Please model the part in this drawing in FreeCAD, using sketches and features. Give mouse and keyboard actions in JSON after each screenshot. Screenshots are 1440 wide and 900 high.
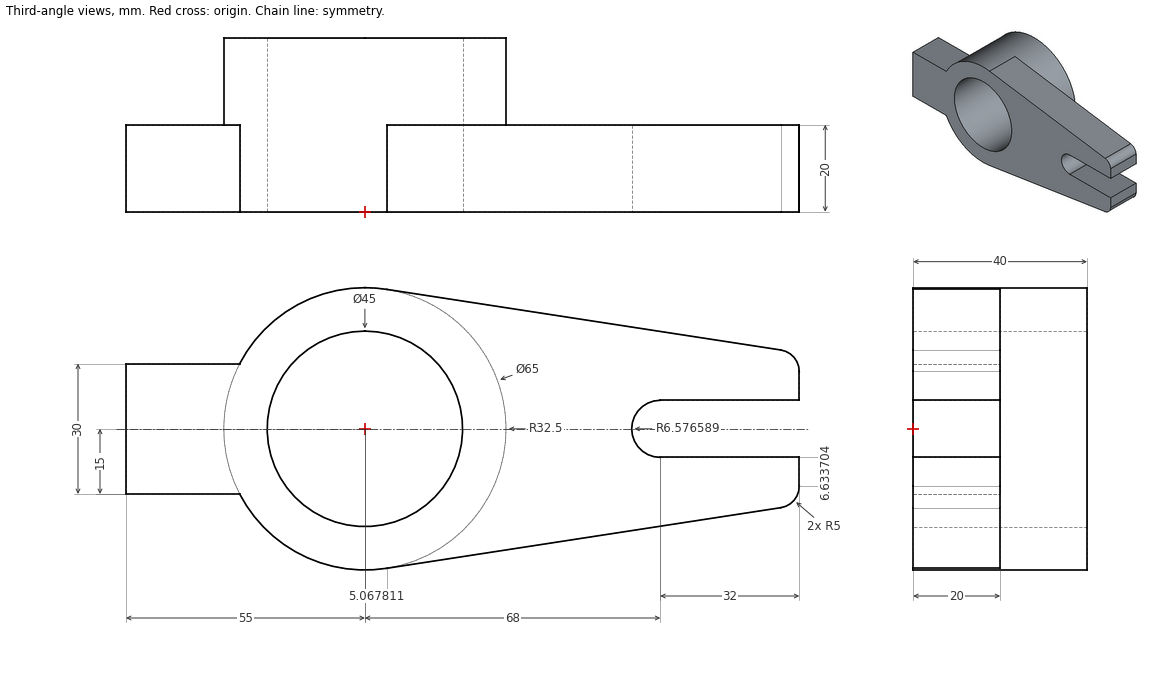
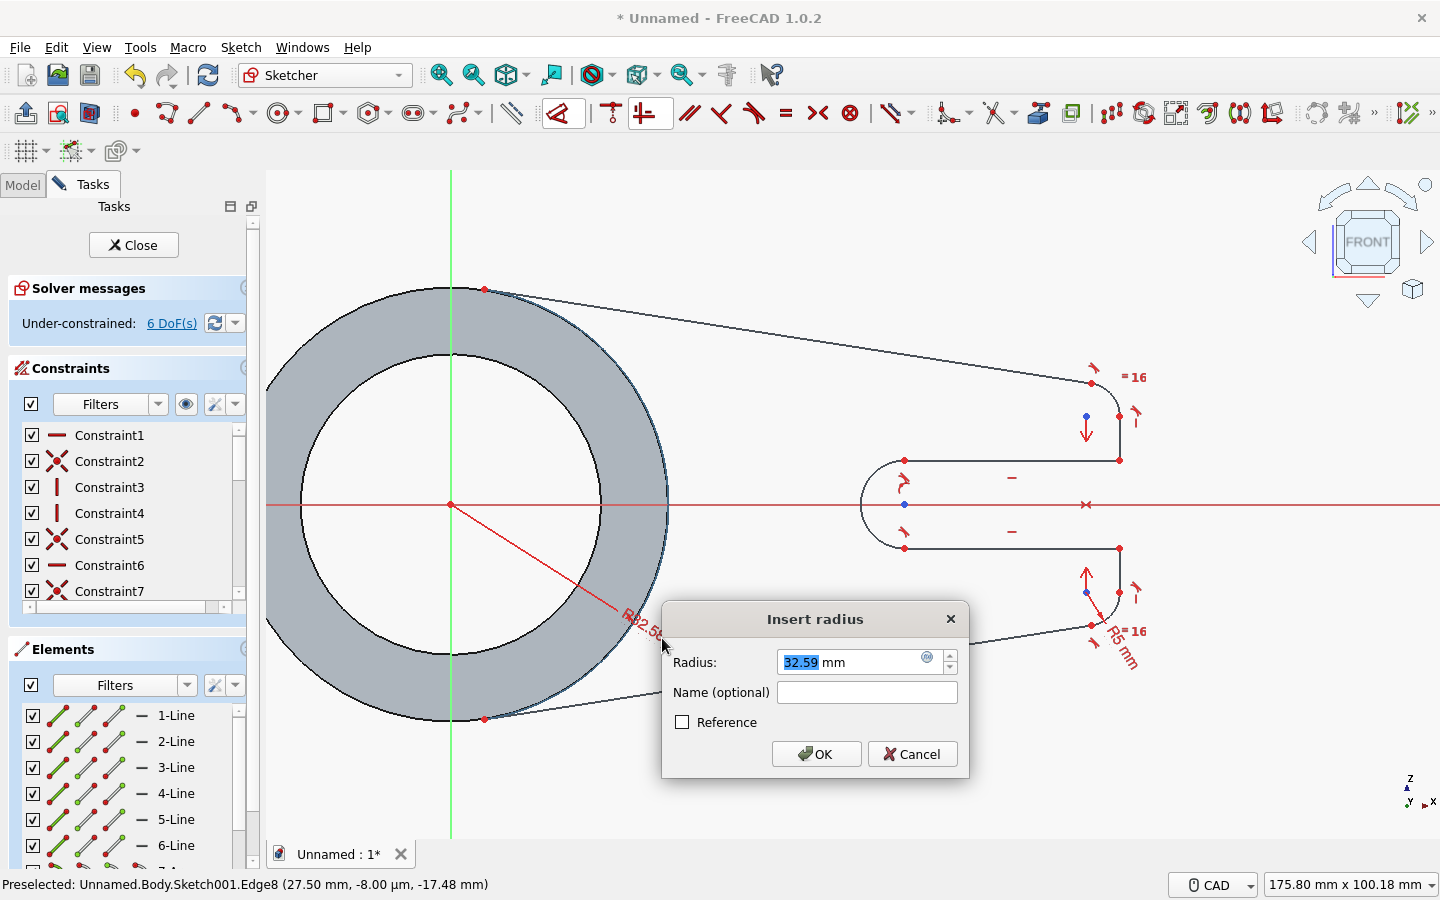
{"action": "type", "text": "32.5"}
{"action": "key", "text": "Return"}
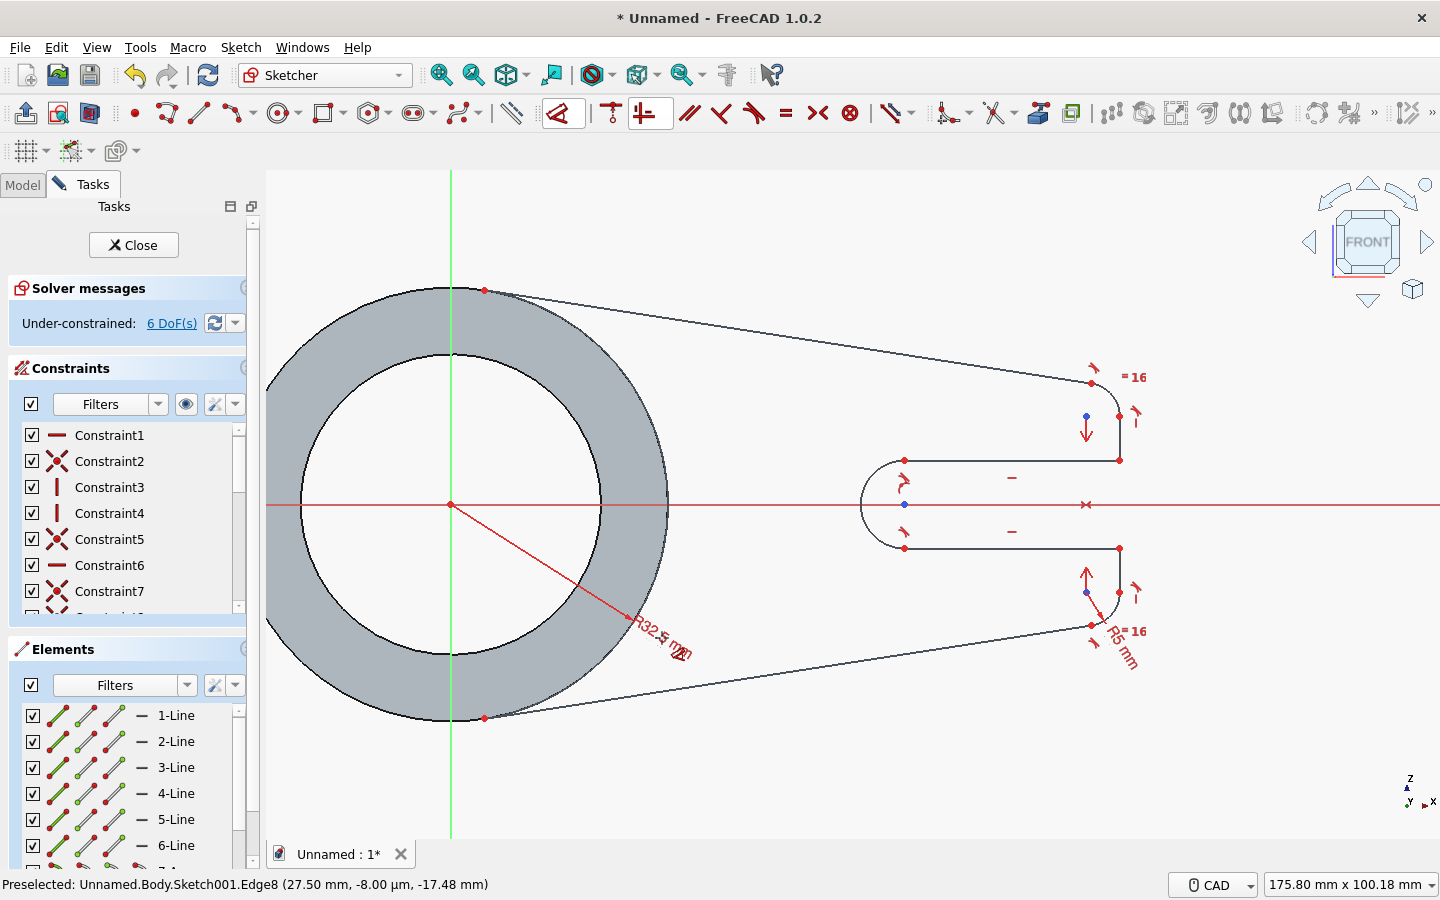
{"action": "left_click", "coordinate": [869, 479]}
{"action": "left_click", "coordinate": [843, 460]}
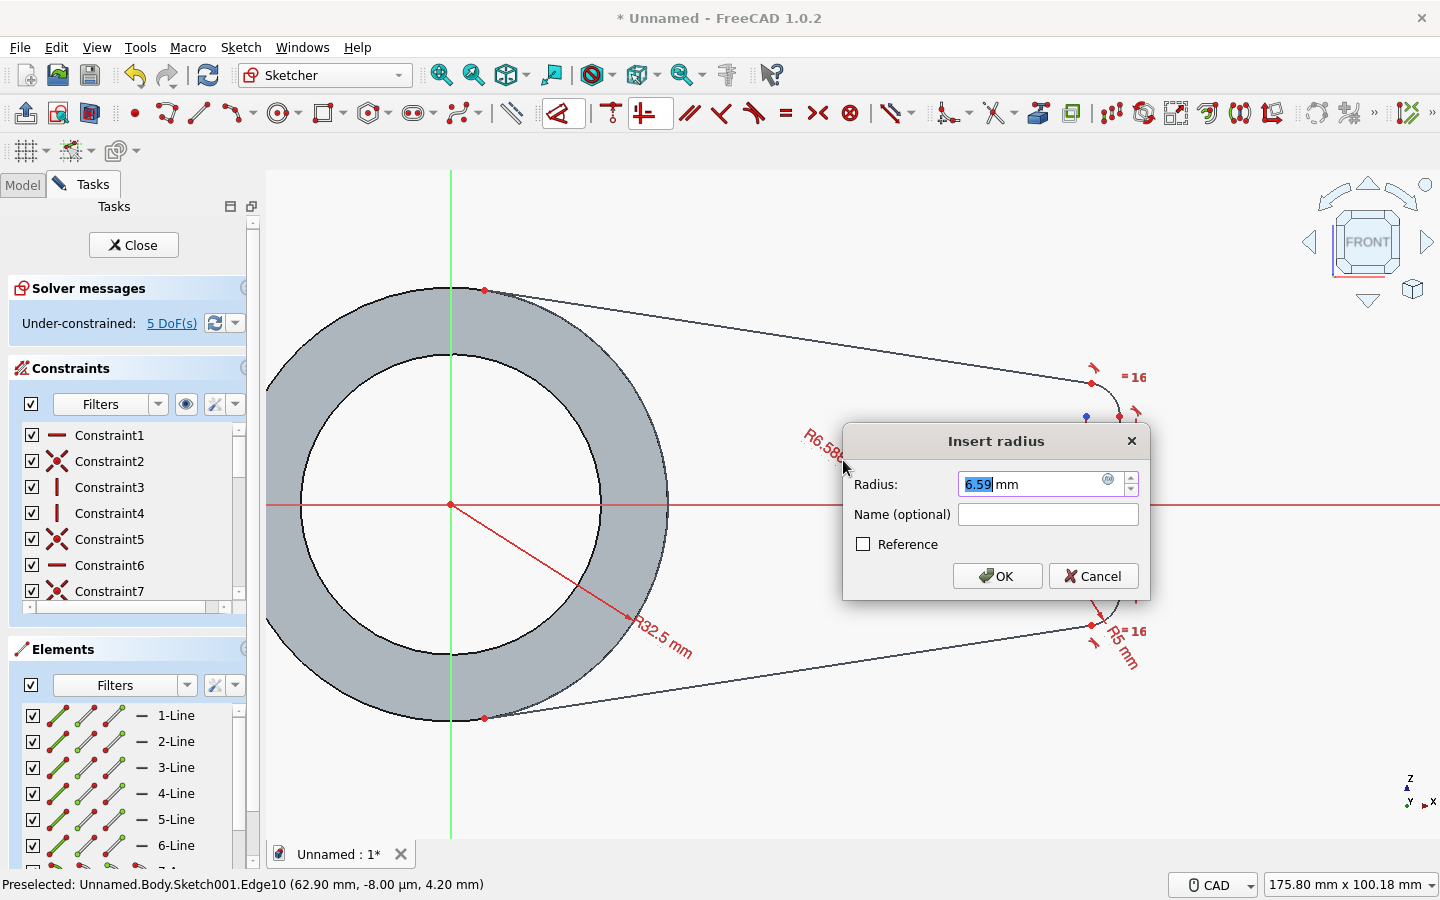
{"action": "type", "text": "6.576589"}
{"action": "key", "text": "Return"}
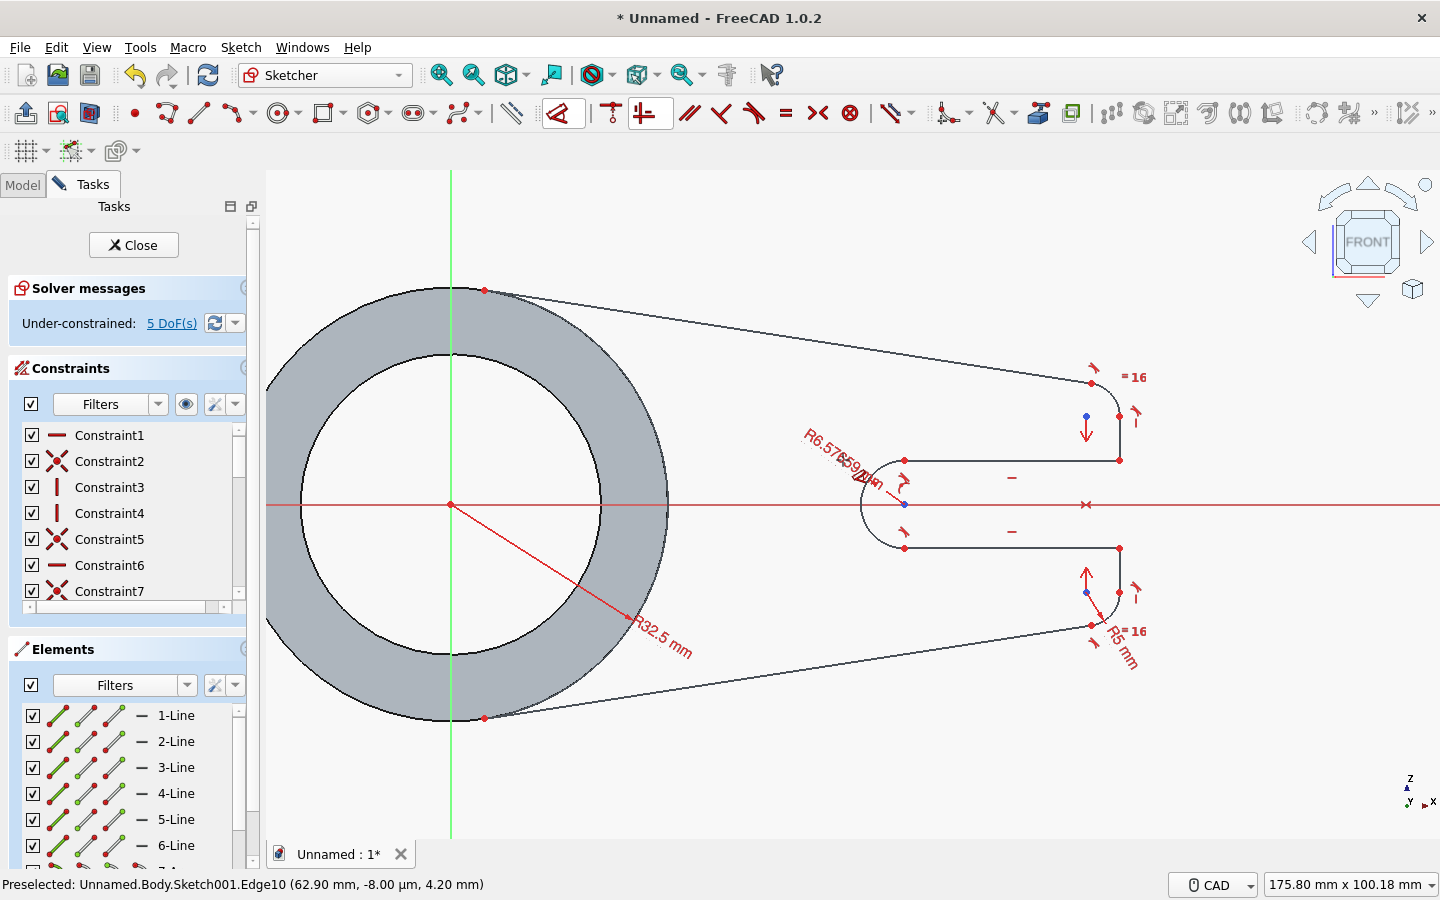
{"action": "left_click", "coordinate": [969, 548]}
{"action": "left_click", "coordinate": [1012, 582]}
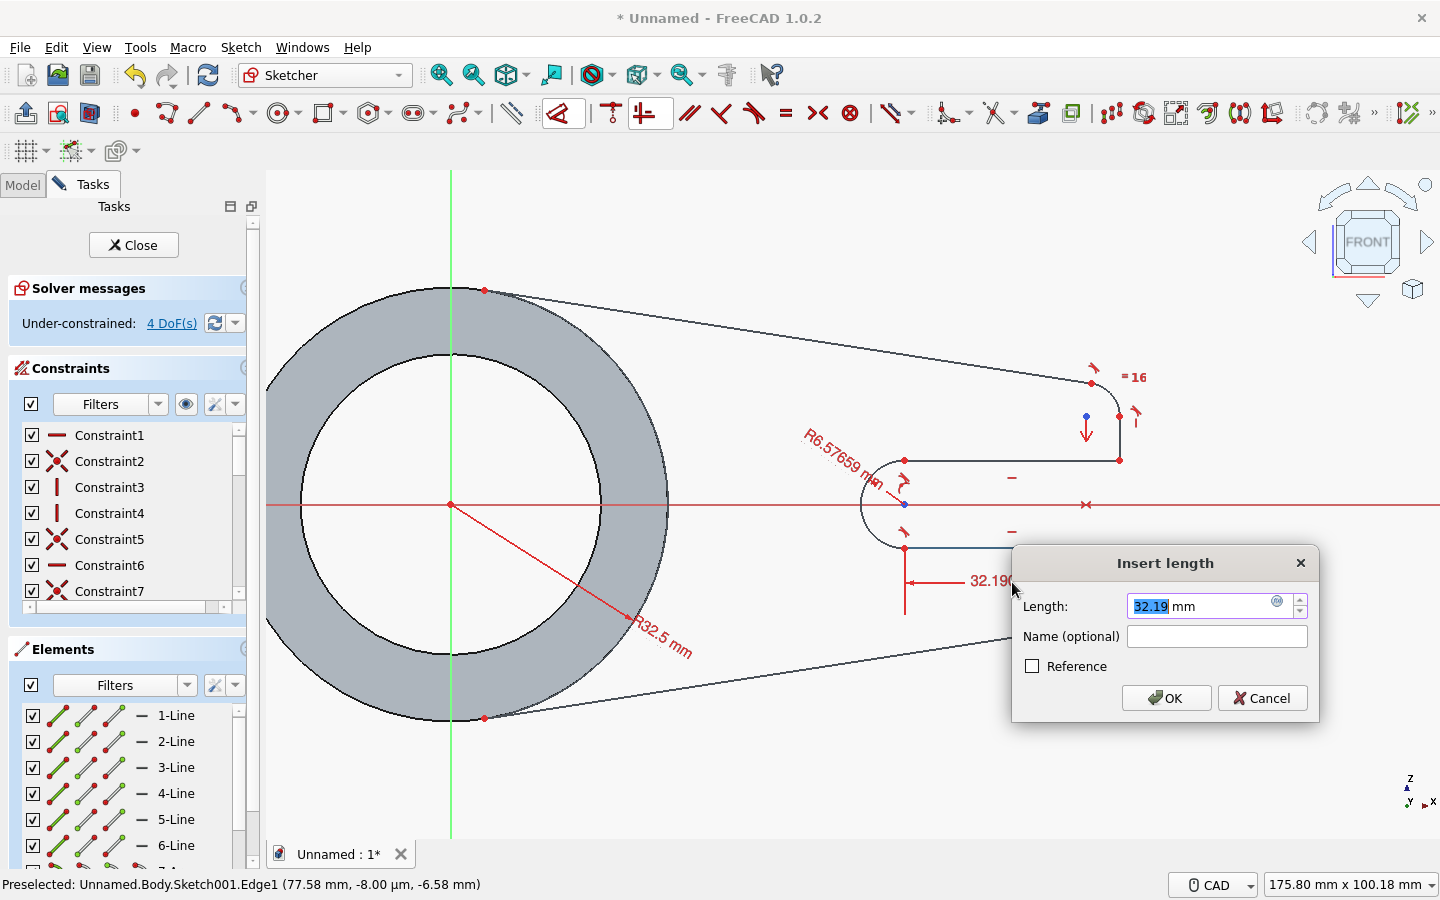
{"action": "type", "text": "32"}
{"action": "key", "text": "Return"}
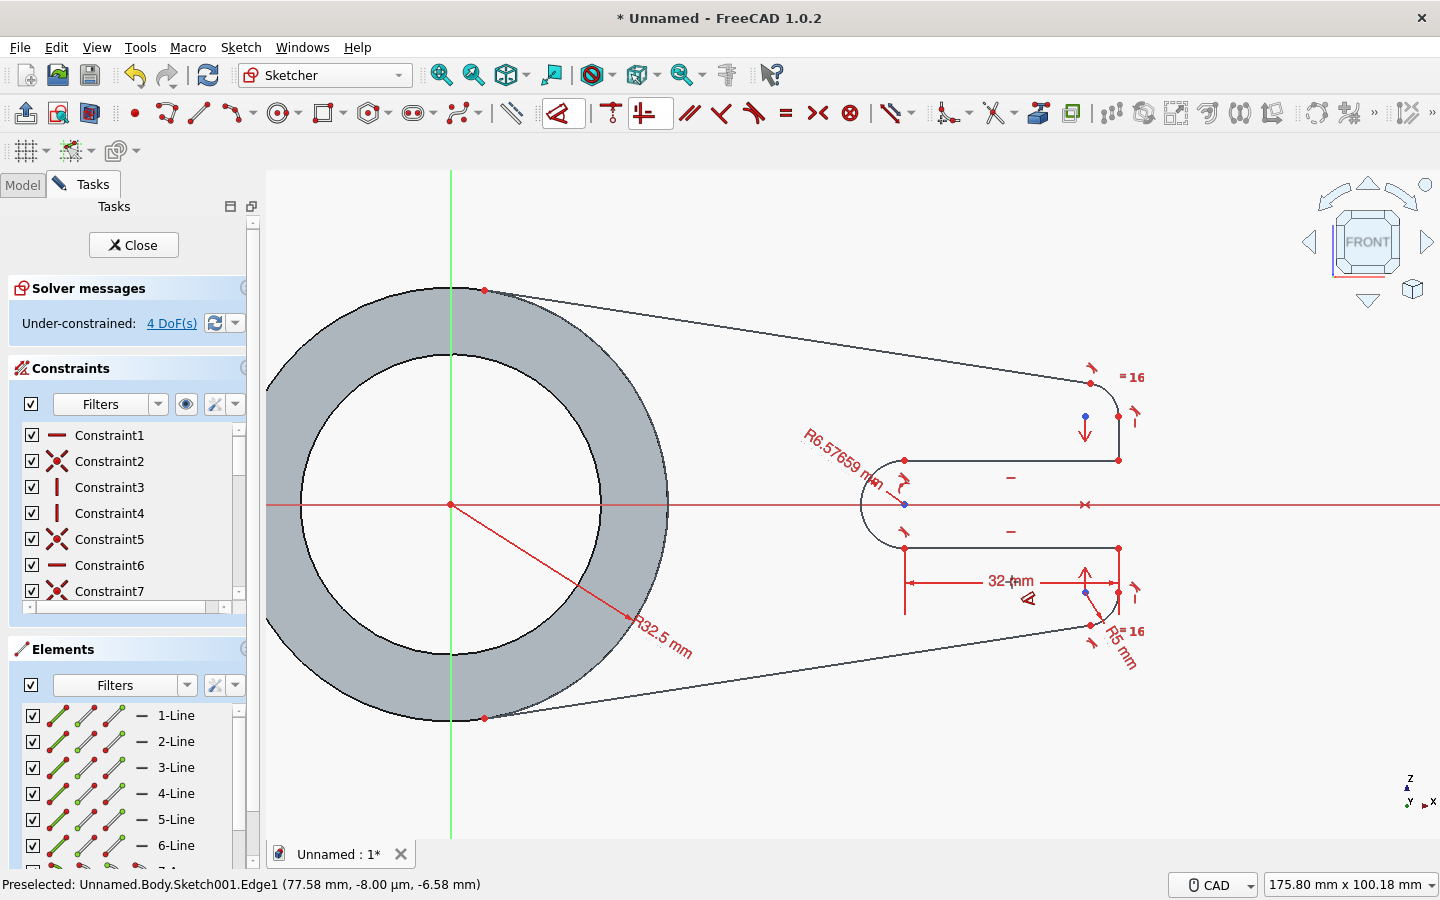
{"action": "left_click", "coordinate": [905, 548]}
{"action": "left_click", "coordinate": [678, 582]}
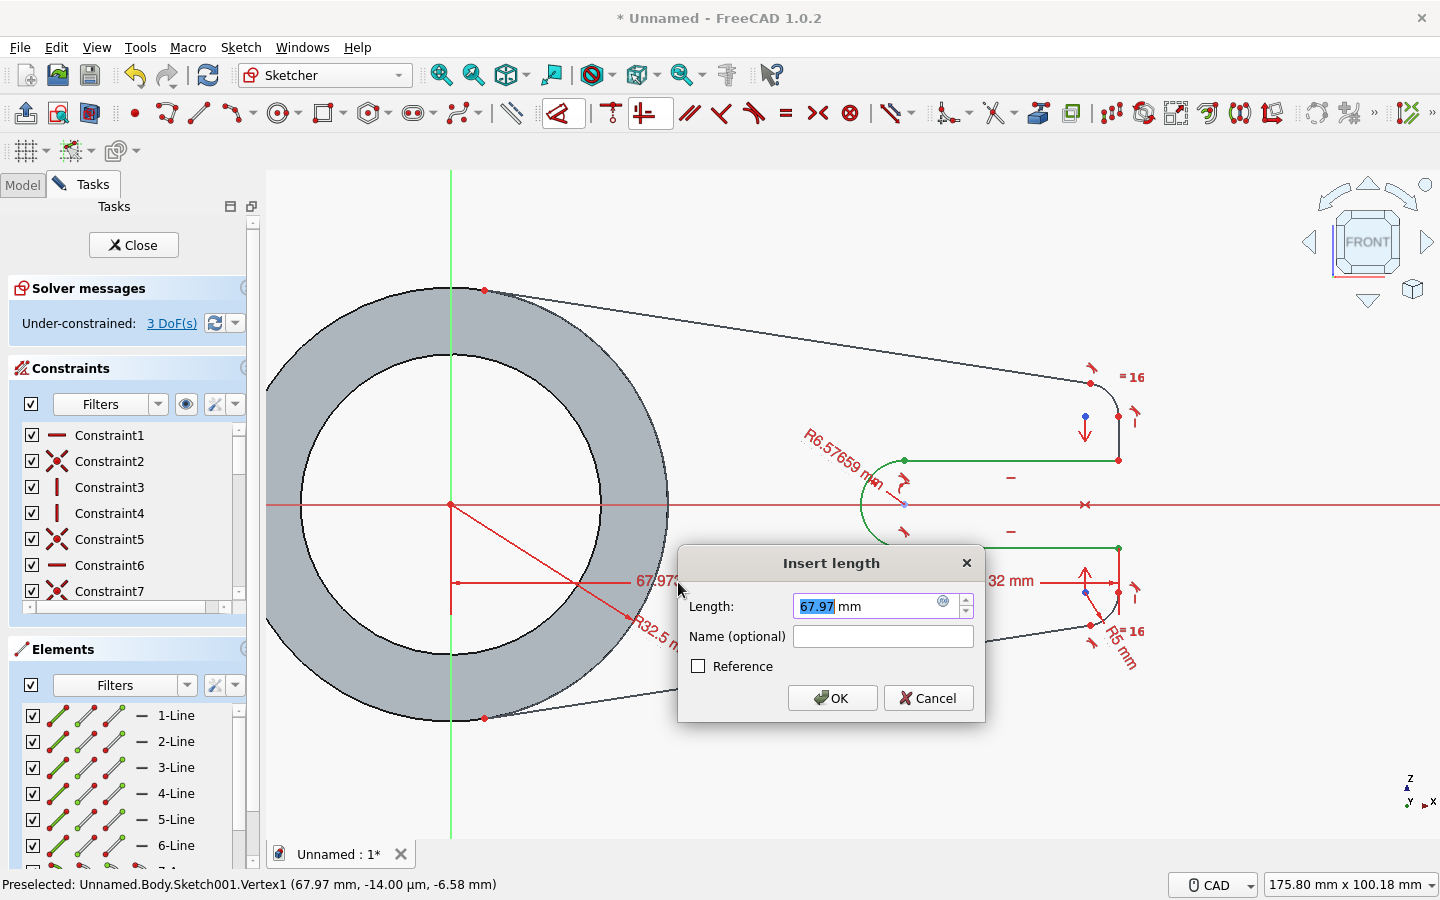
{"action": "type", "text": "68"}
{"action": "key", "text": "Return"}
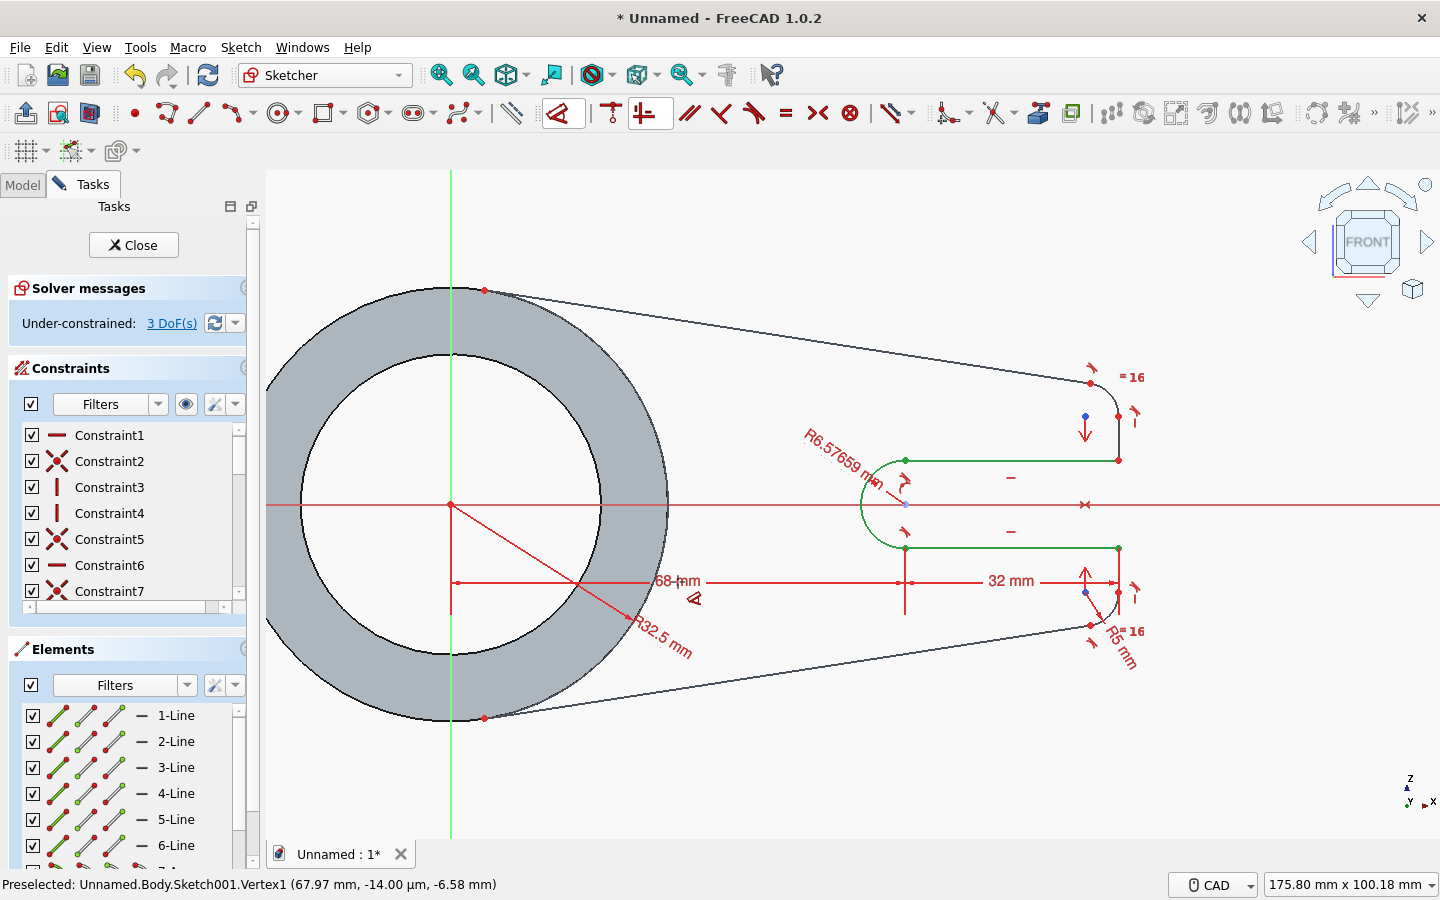
{"action": "left_click", "coordinate": [1119, 562]}
{"action": "left_click", "coordinate": [1153, 570]}